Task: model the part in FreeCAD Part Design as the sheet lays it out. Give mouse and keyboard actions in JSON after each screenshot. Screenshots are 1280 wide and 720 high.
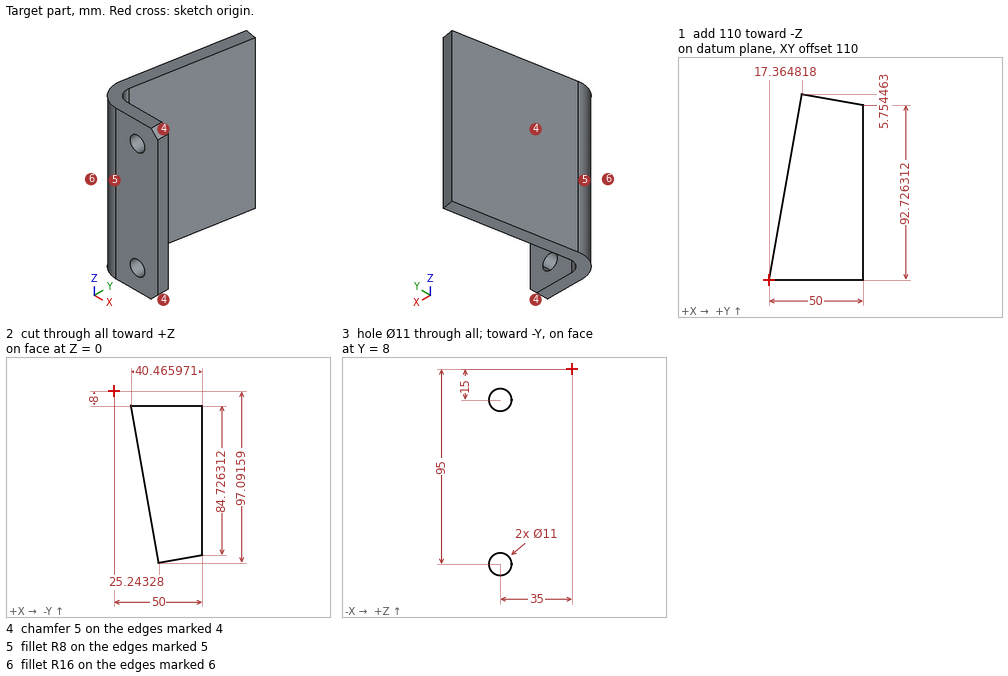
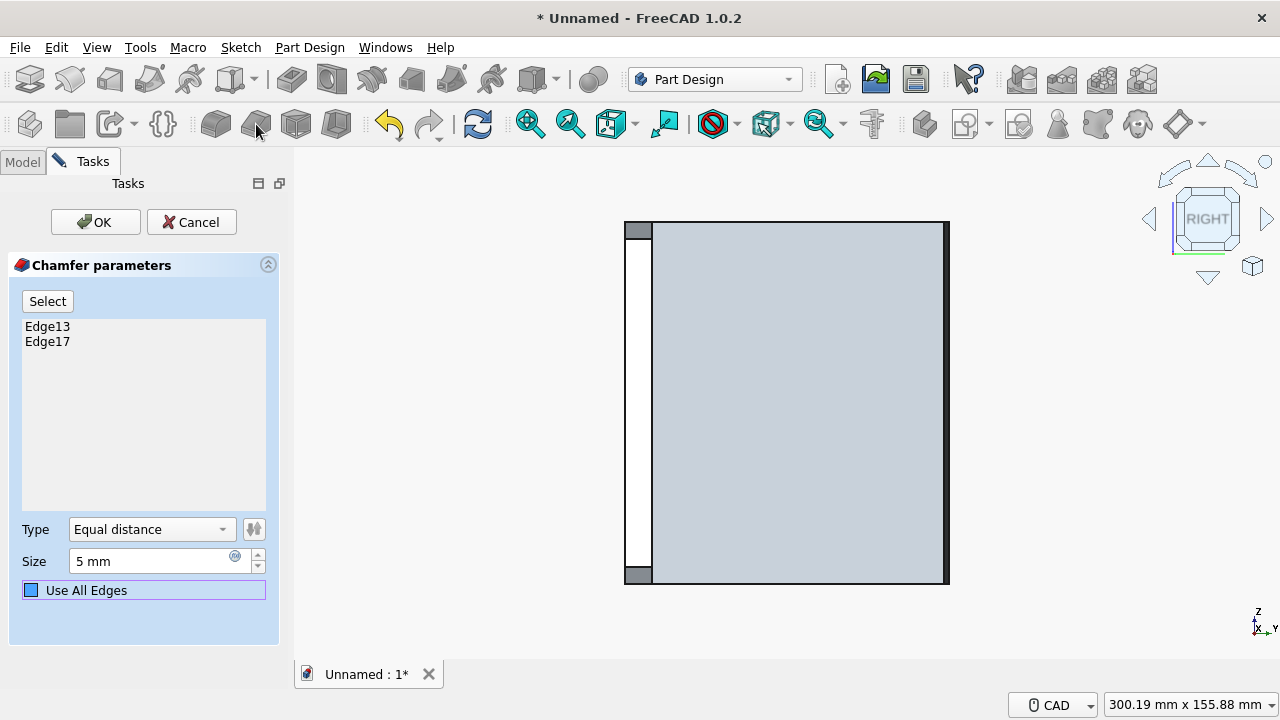
{"action": "left_click", "coordinate": [96, 222]}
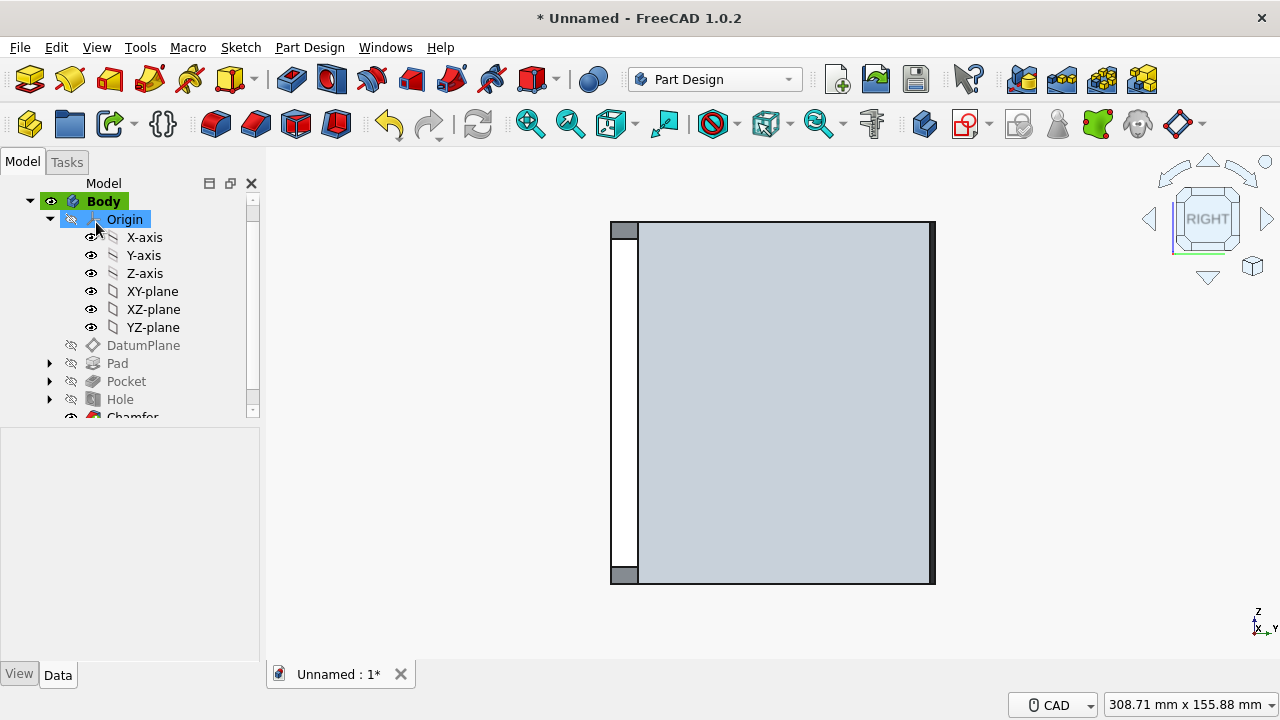
{"action": "key", "text": "0"}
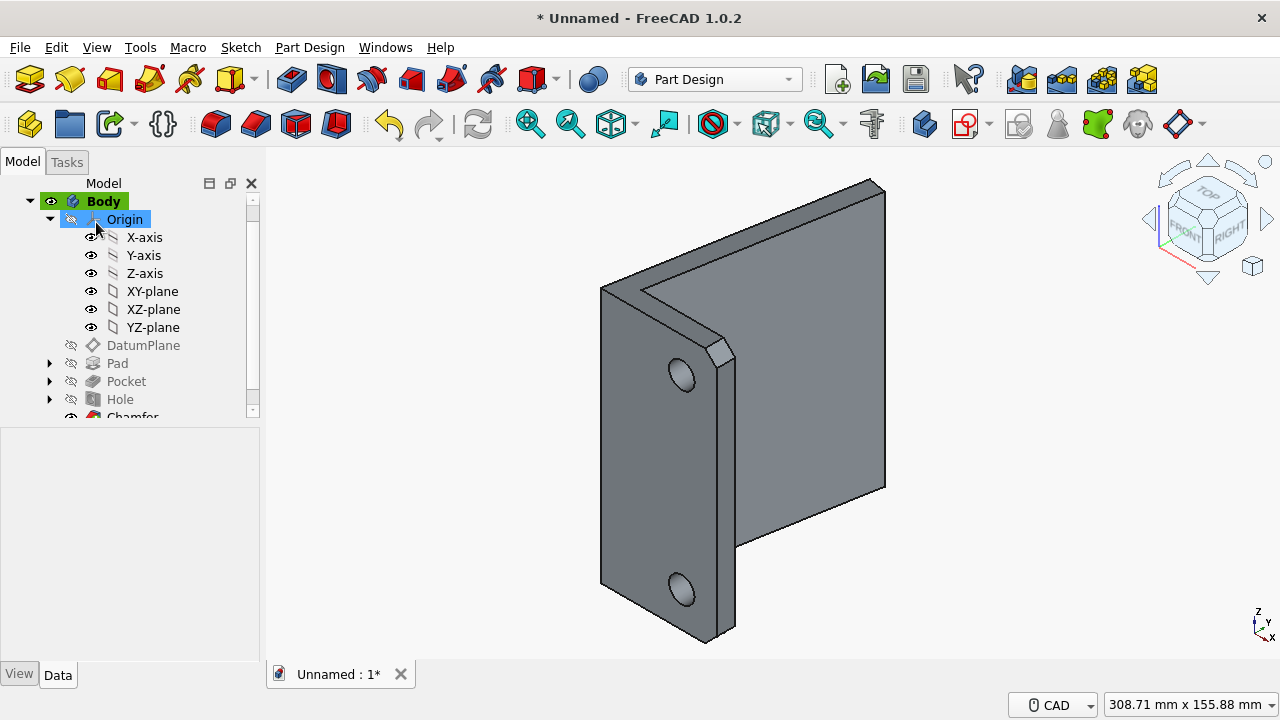
{"action": "key", "text": "2"}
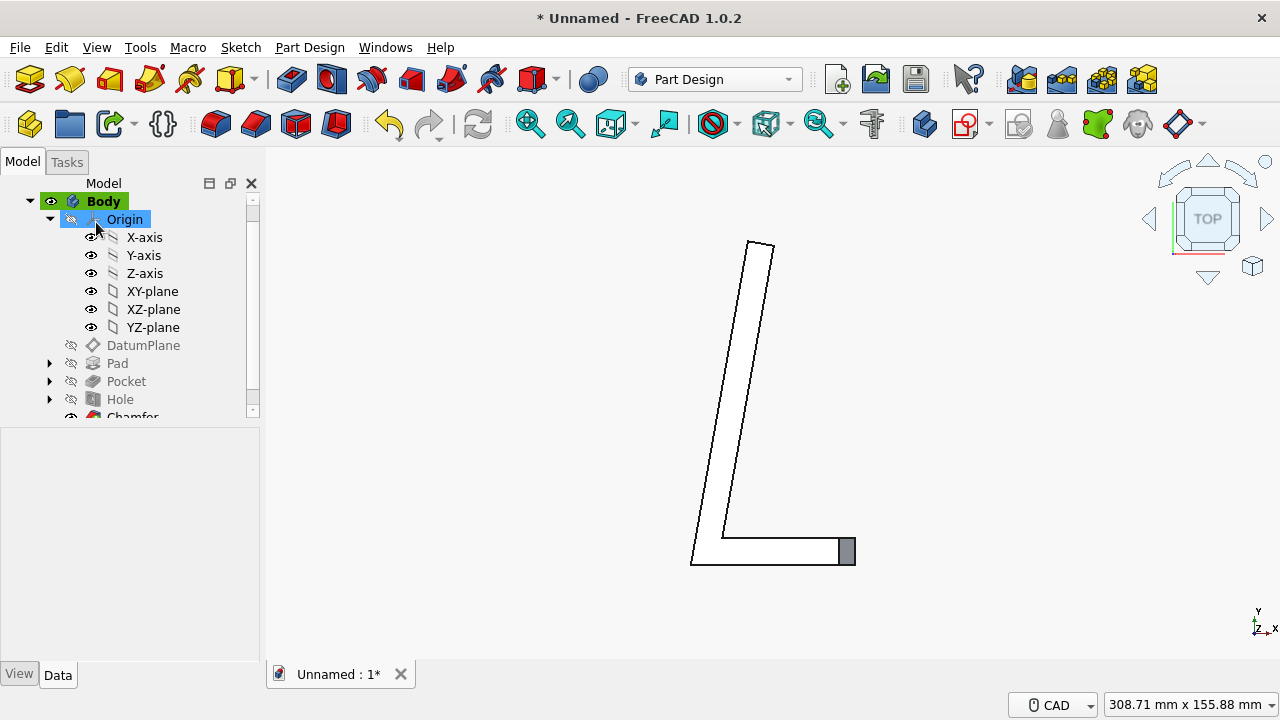
{"action": "key", "text": "1"}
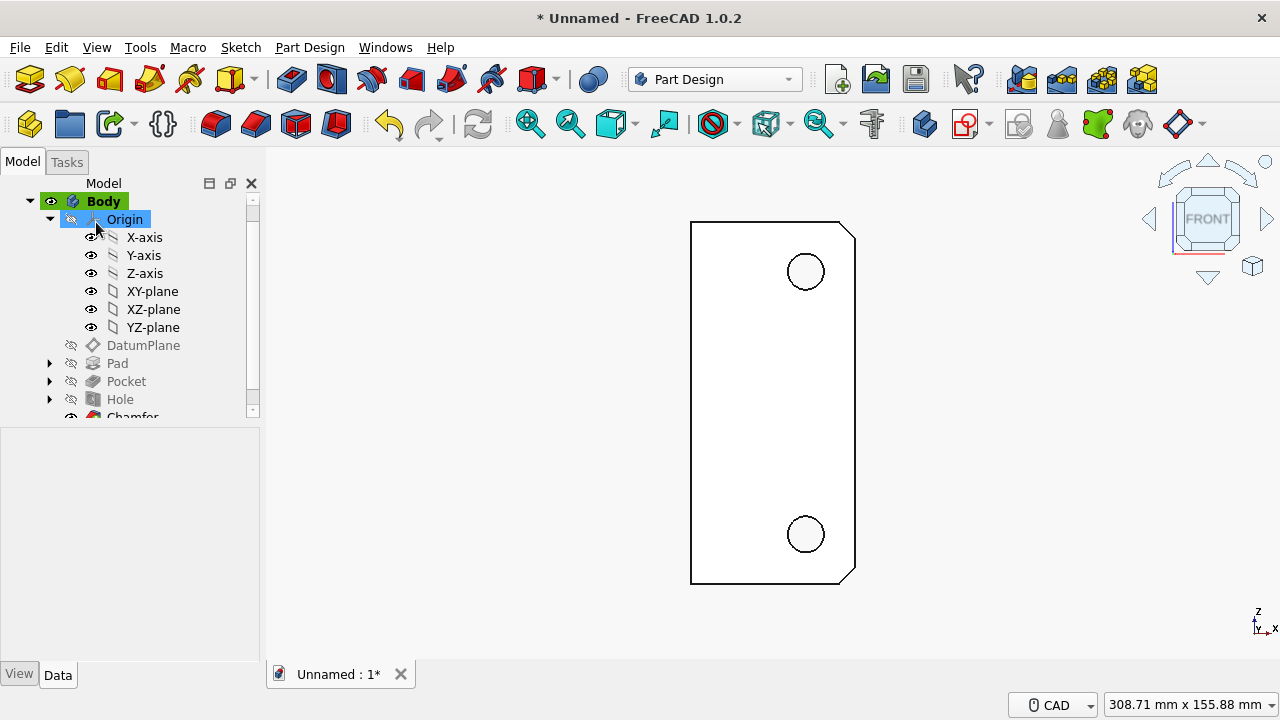
{"action": "key", "text": "3"}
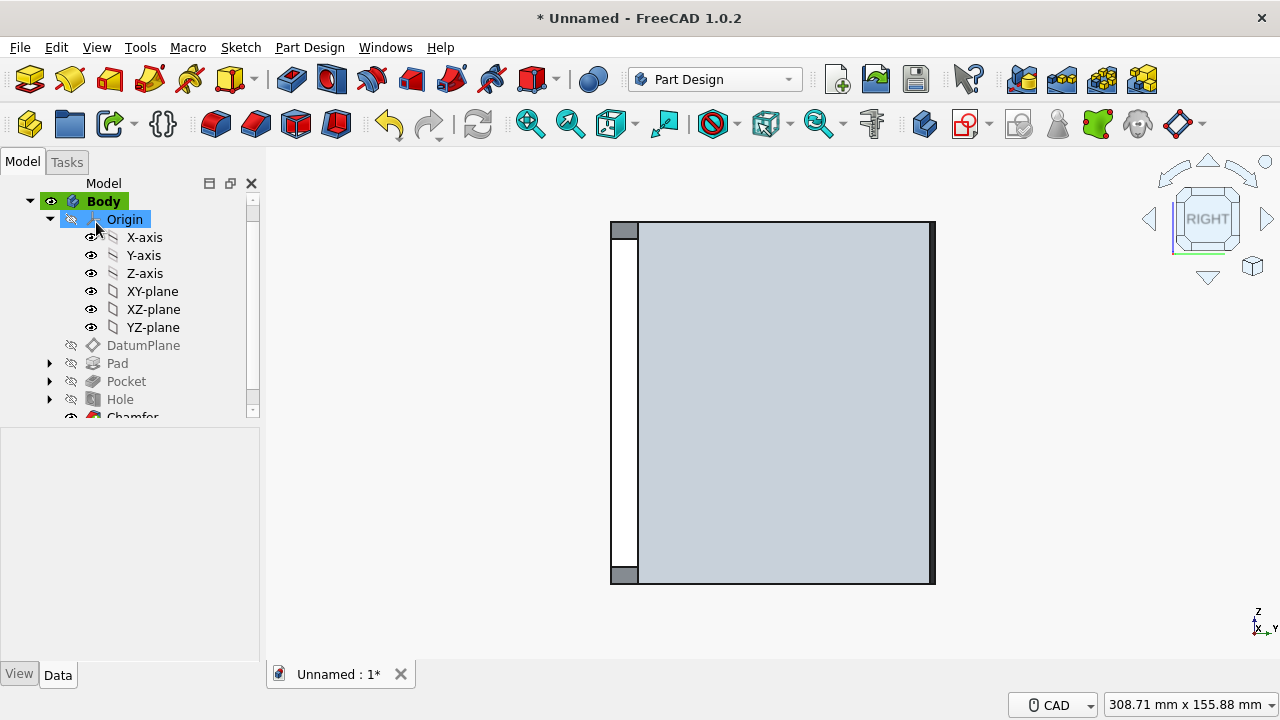
{"action": "key", "text": "5"}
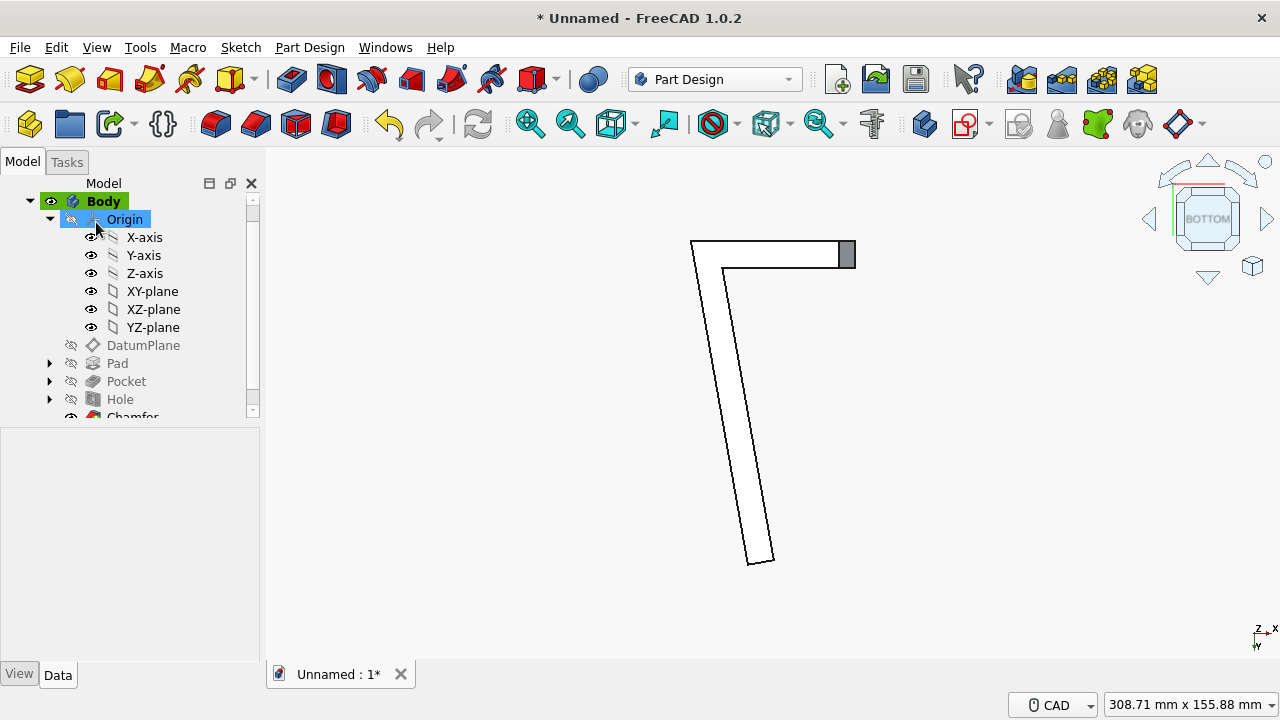
{"action": "key", "text": "4"}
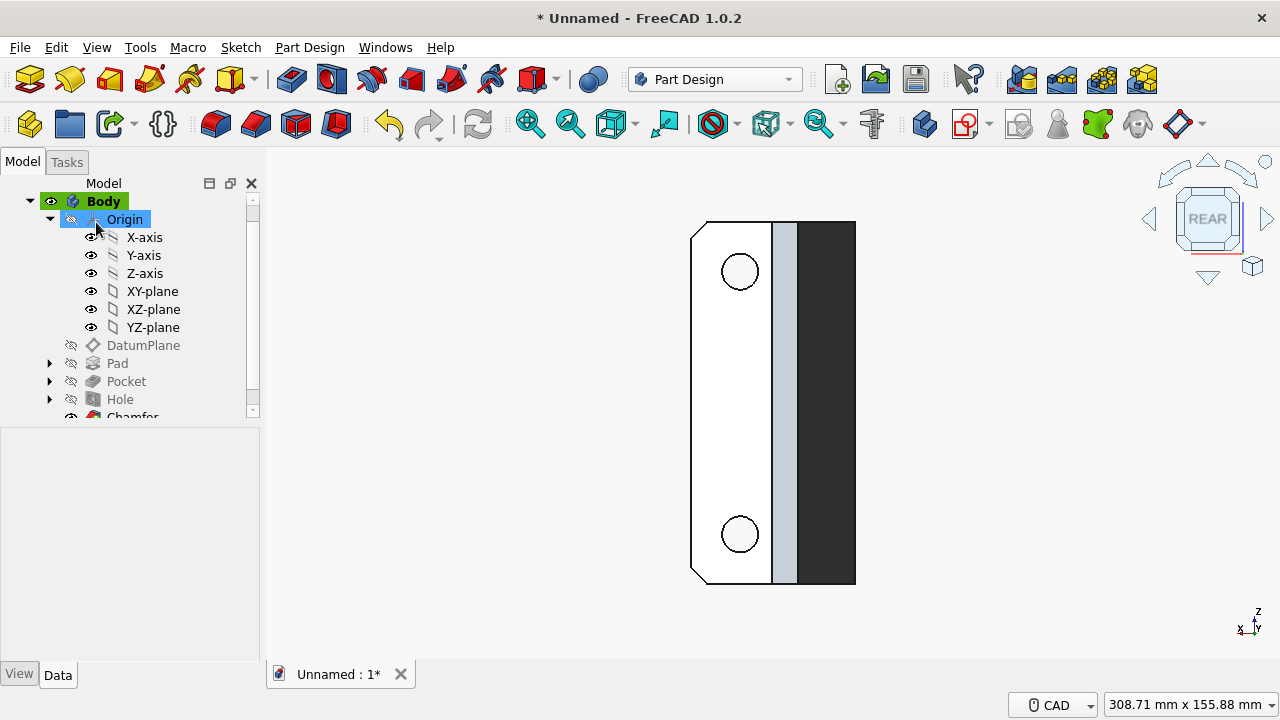
{"action": "key", "text": "6"}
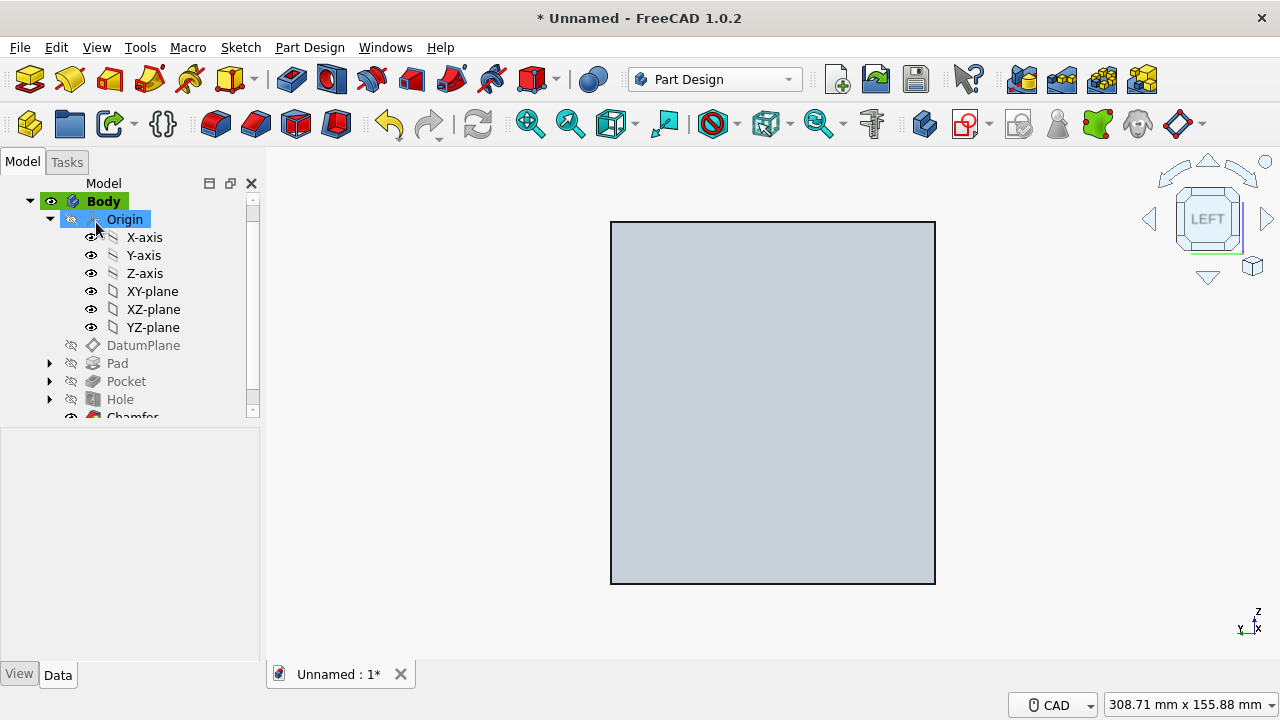
{"action": "key", "text": "v 3"}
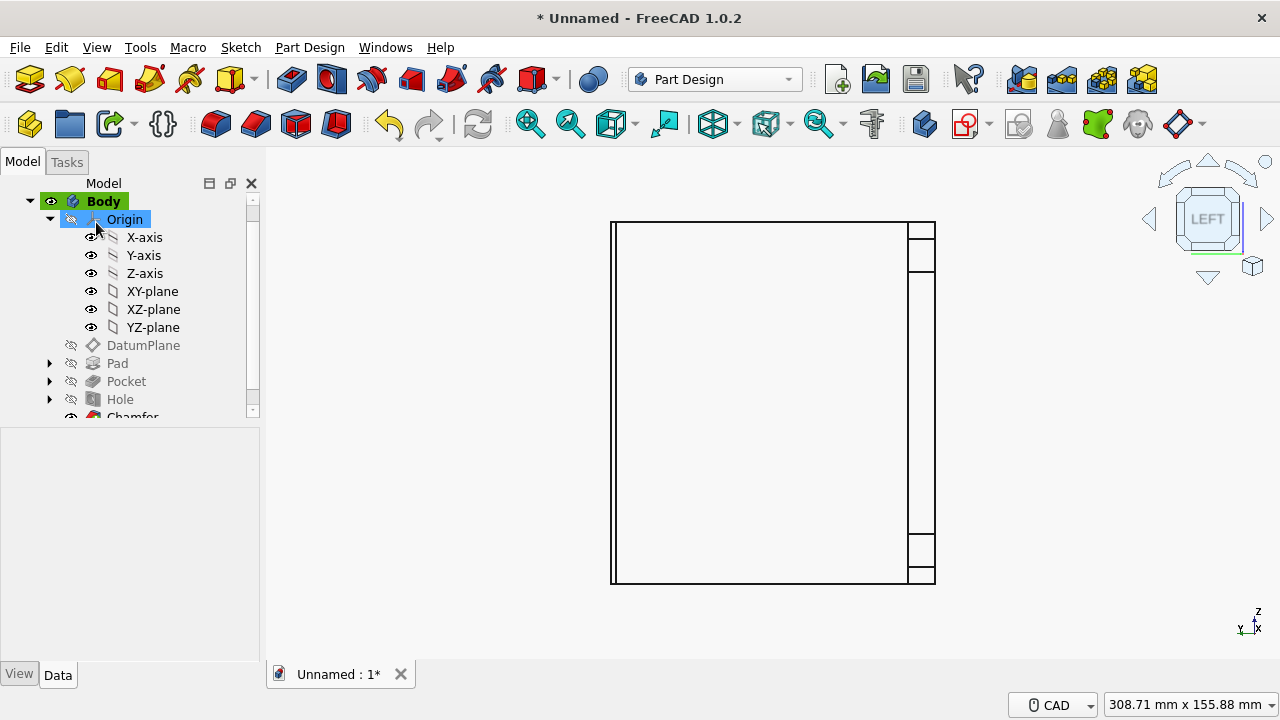
{"action": "key", "text": "0"}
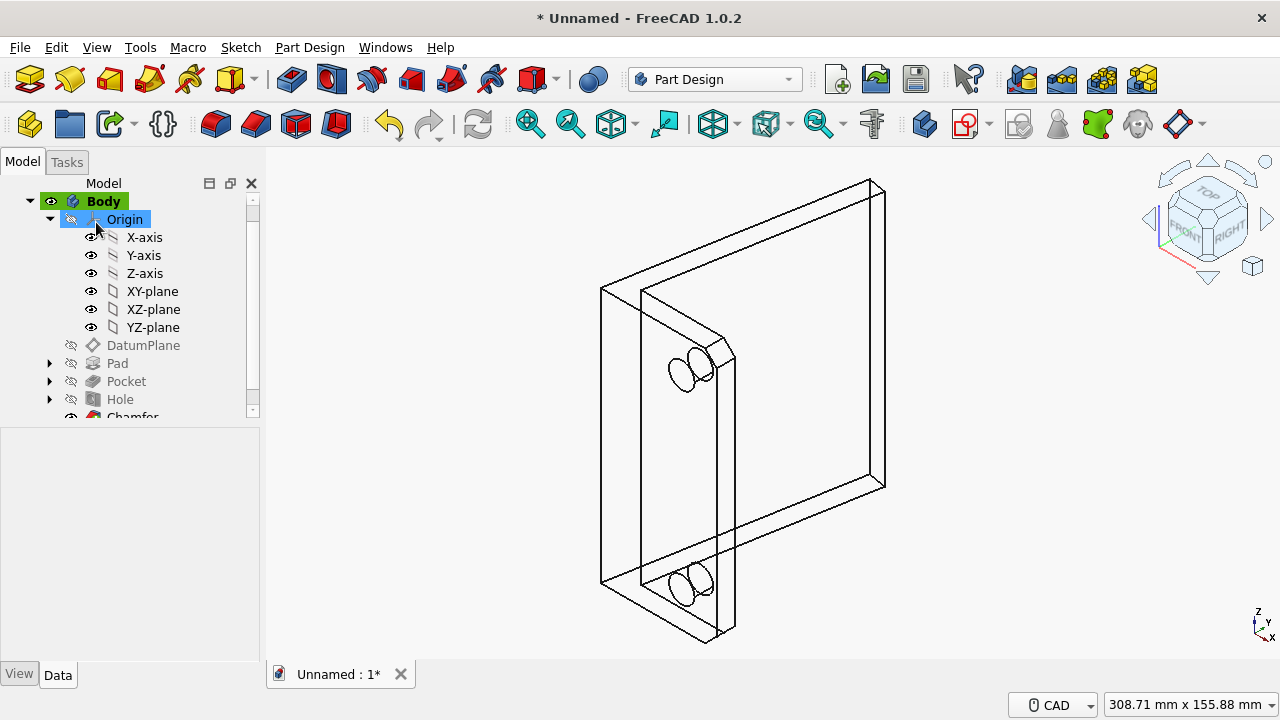
{"action": "left_click", "coordinate": [641, 437]}